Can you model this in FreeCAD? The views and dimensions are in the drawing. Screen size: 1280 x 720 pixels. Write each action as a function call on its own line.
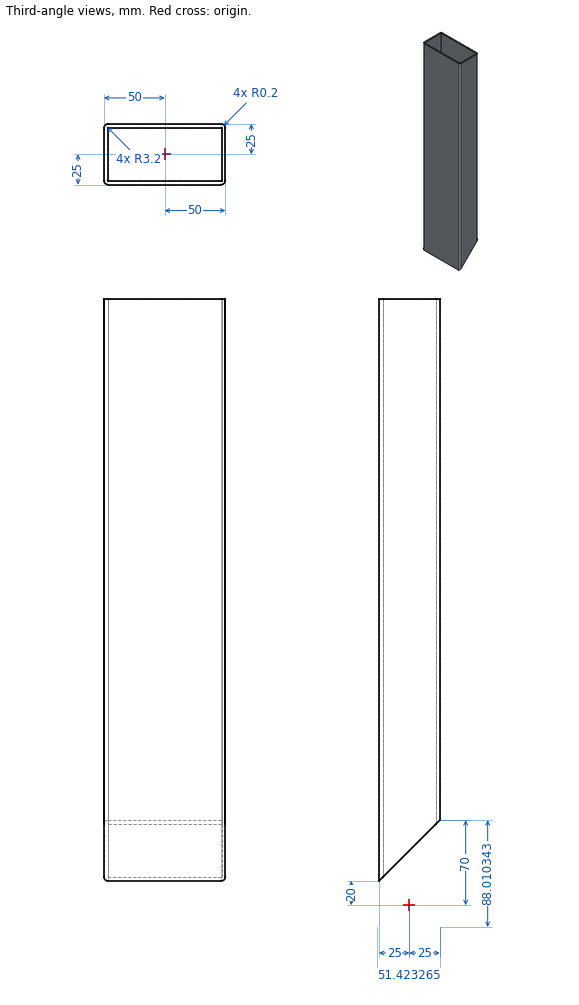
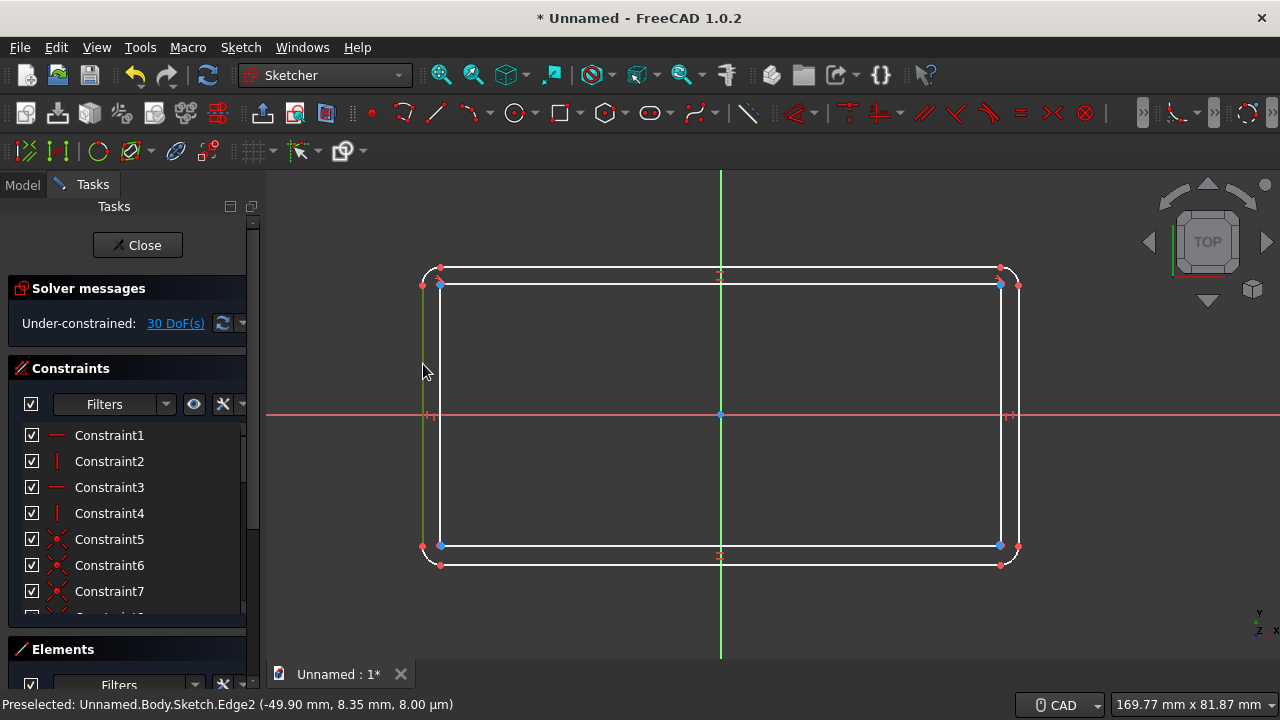
click(428, 272)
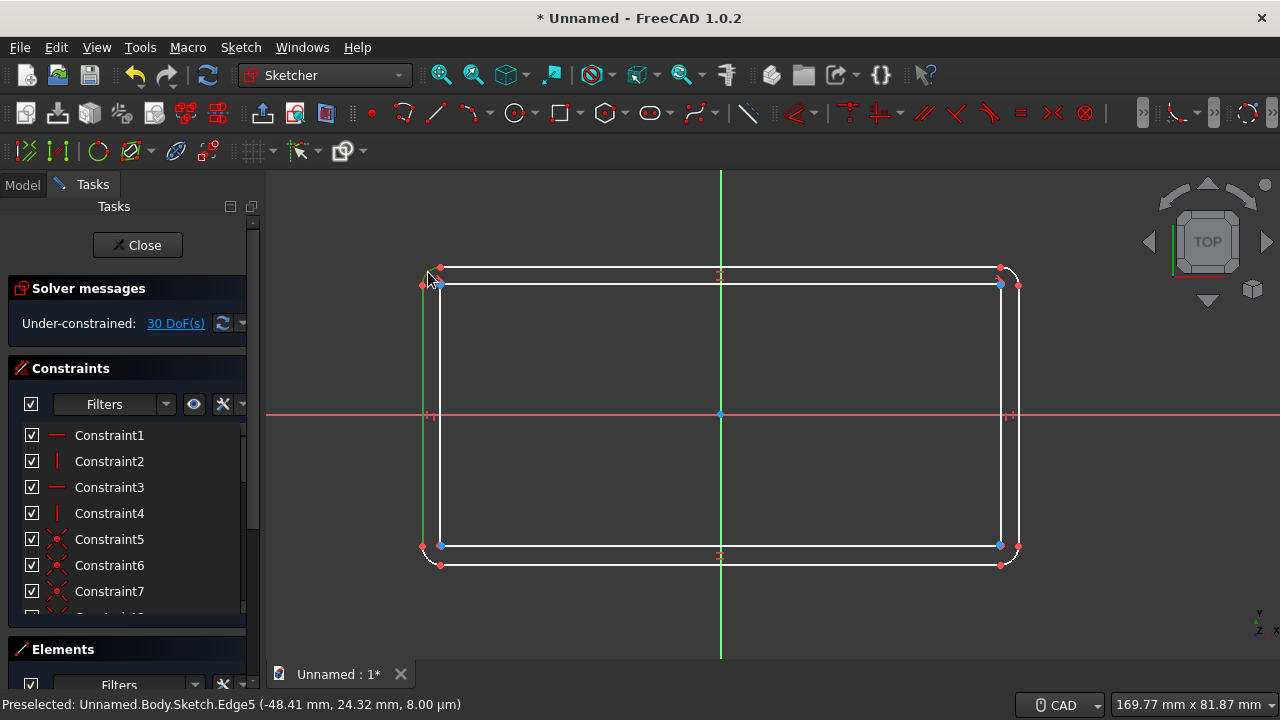
click(990, 114)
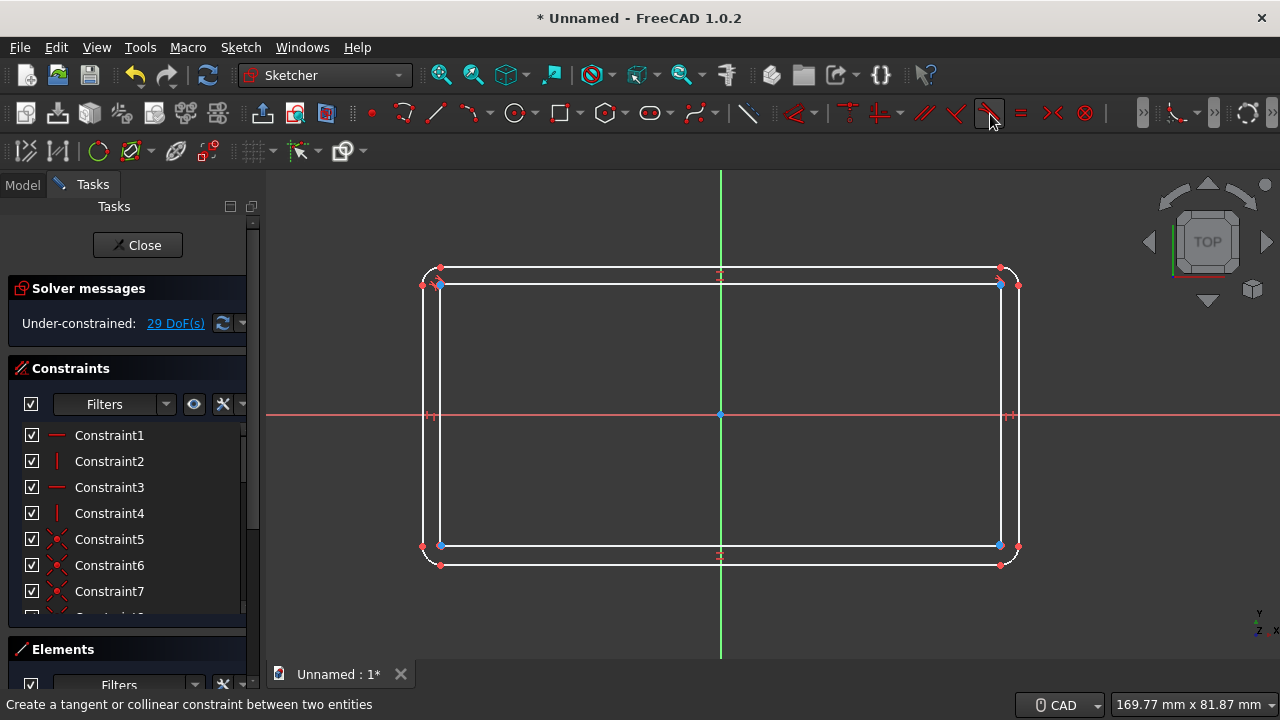
click(423, 364)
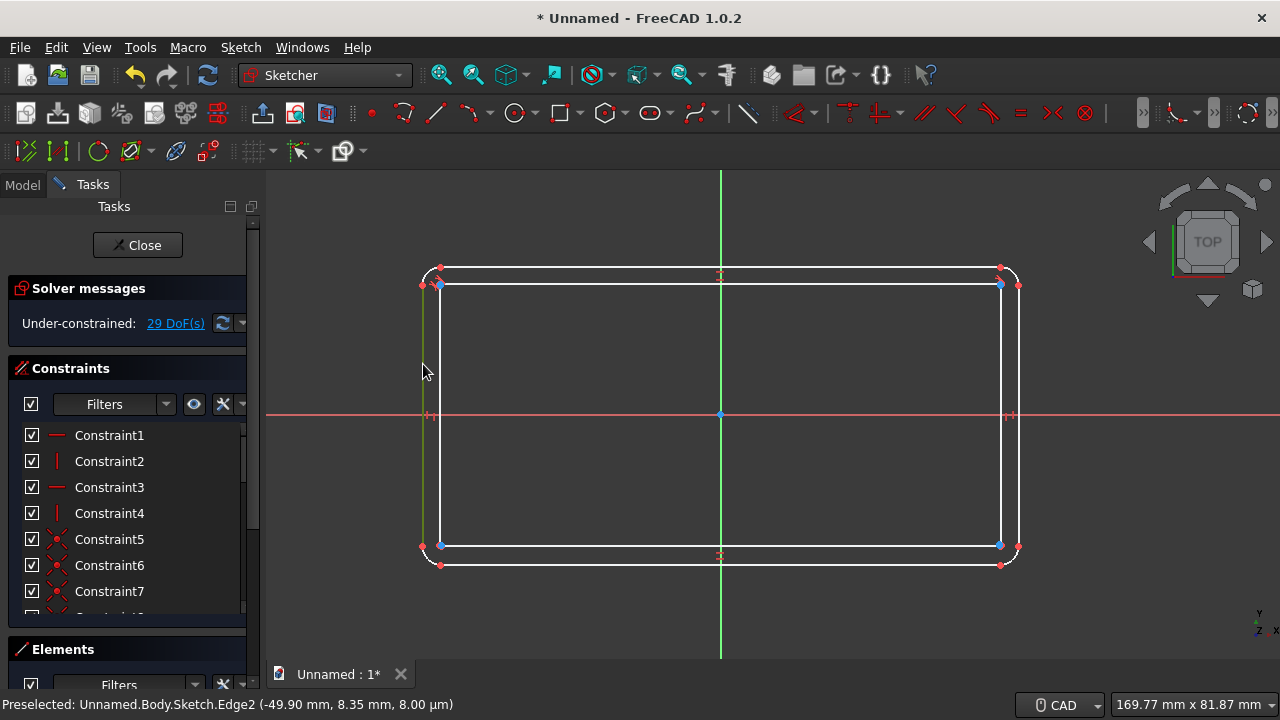
click(428, 559)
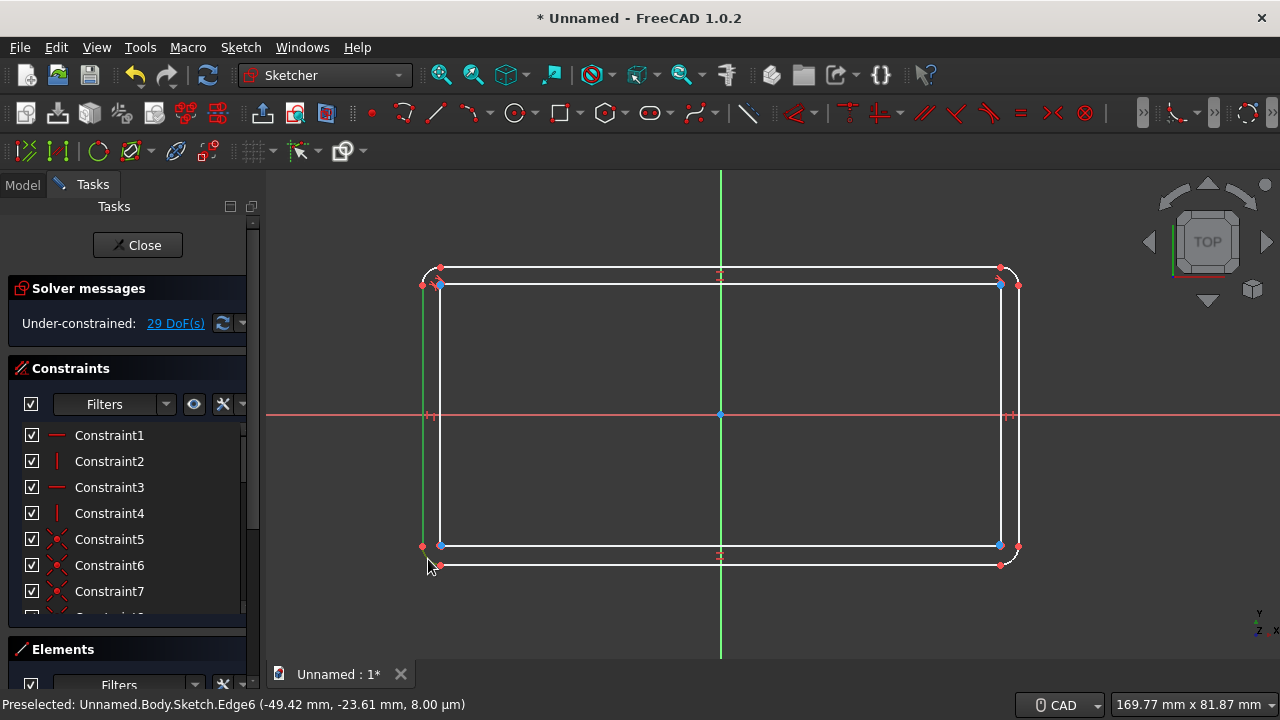
click(990, 114)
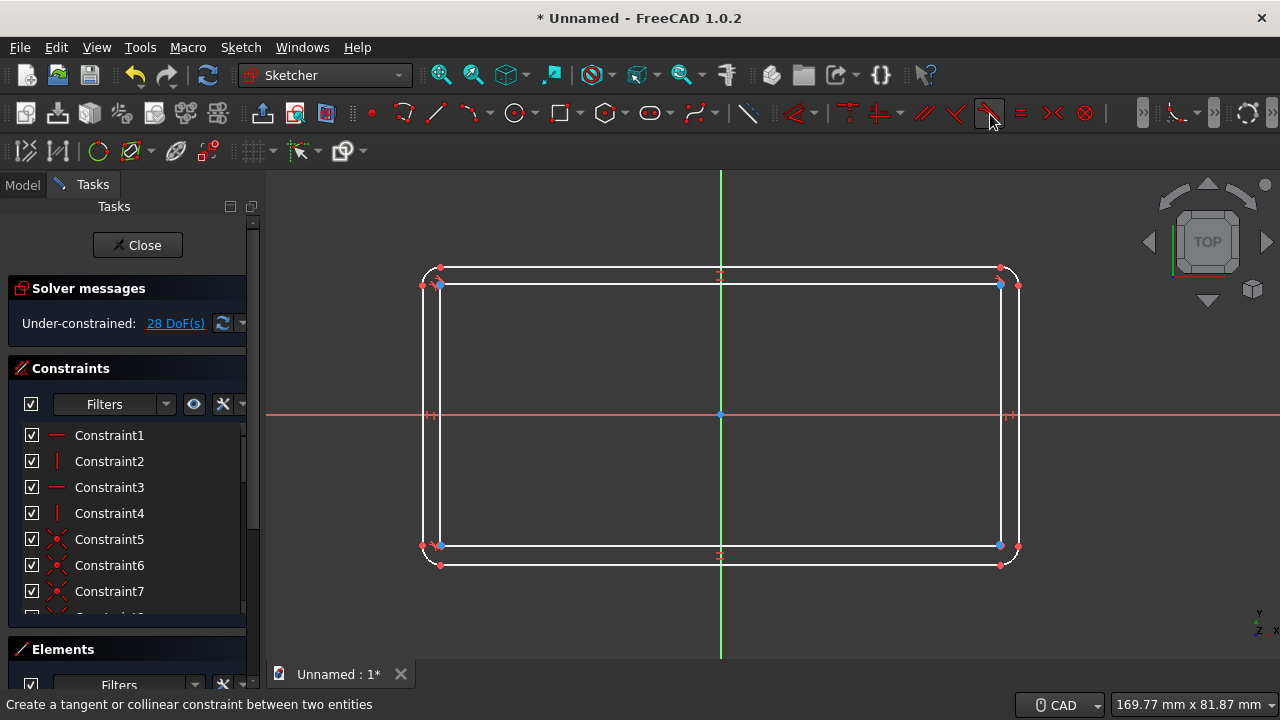
click(609, 565)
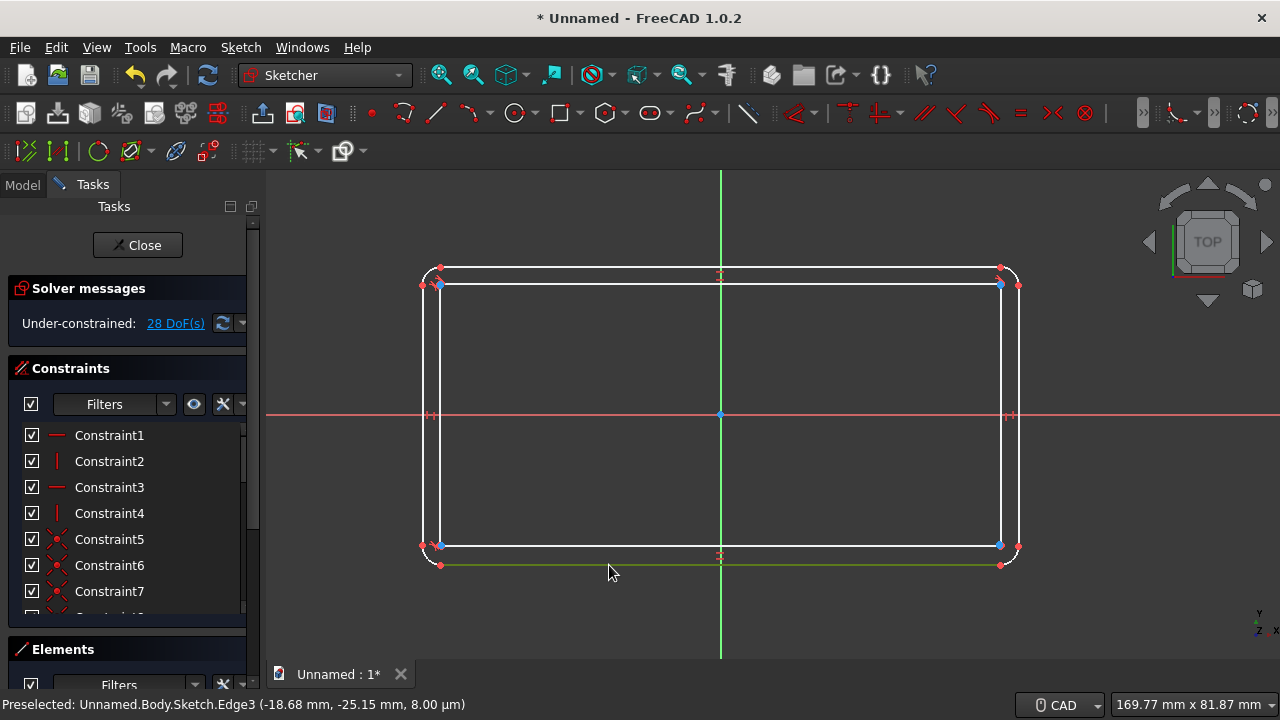
click(428, 559)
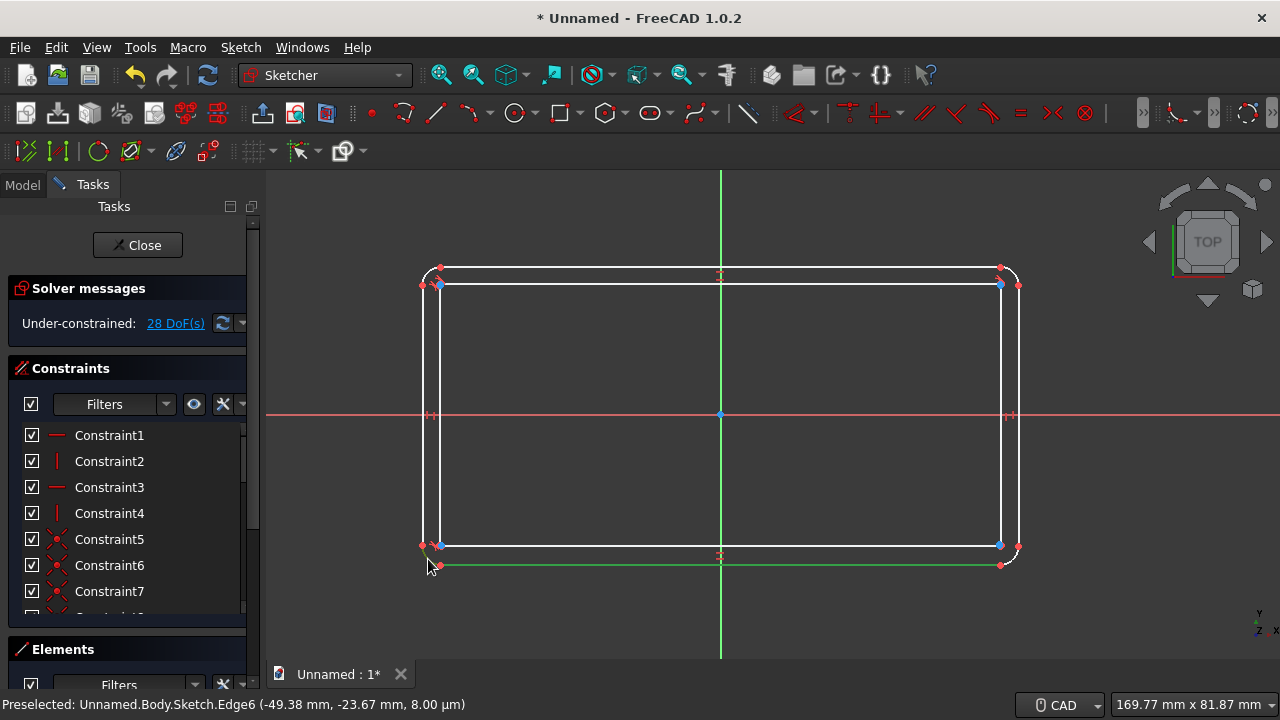
click(990, 114)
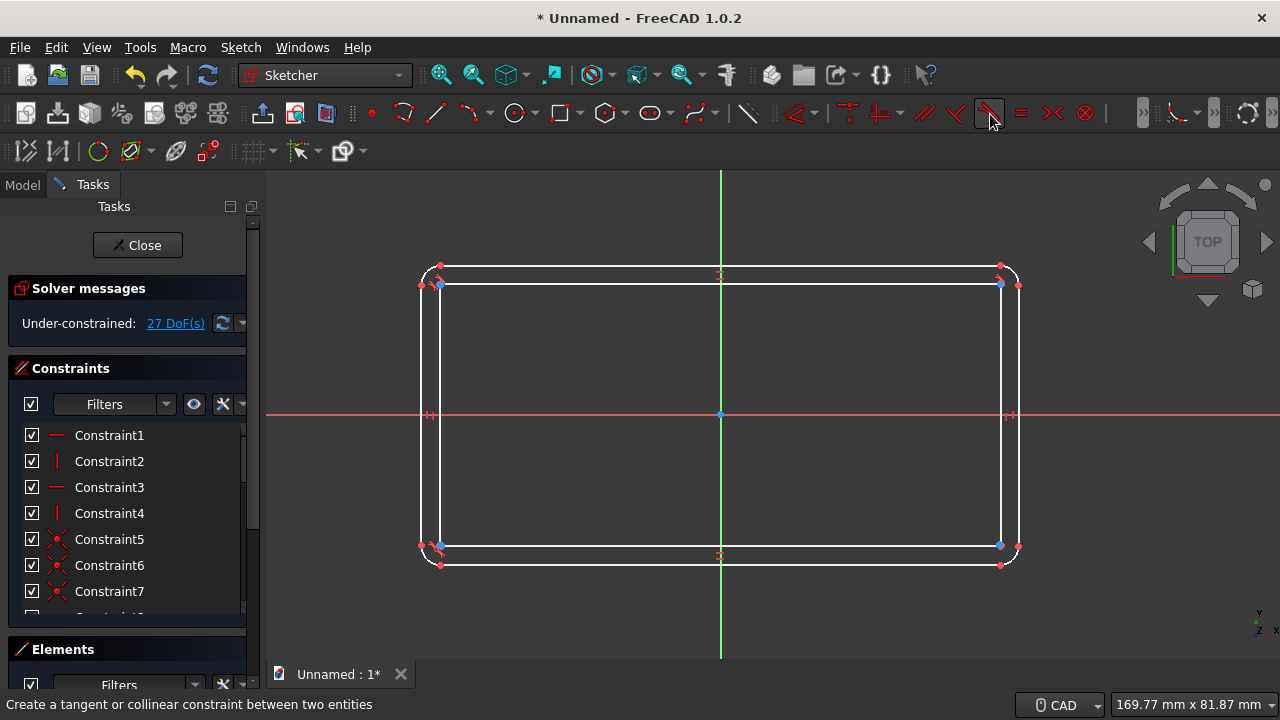
click(609, 565)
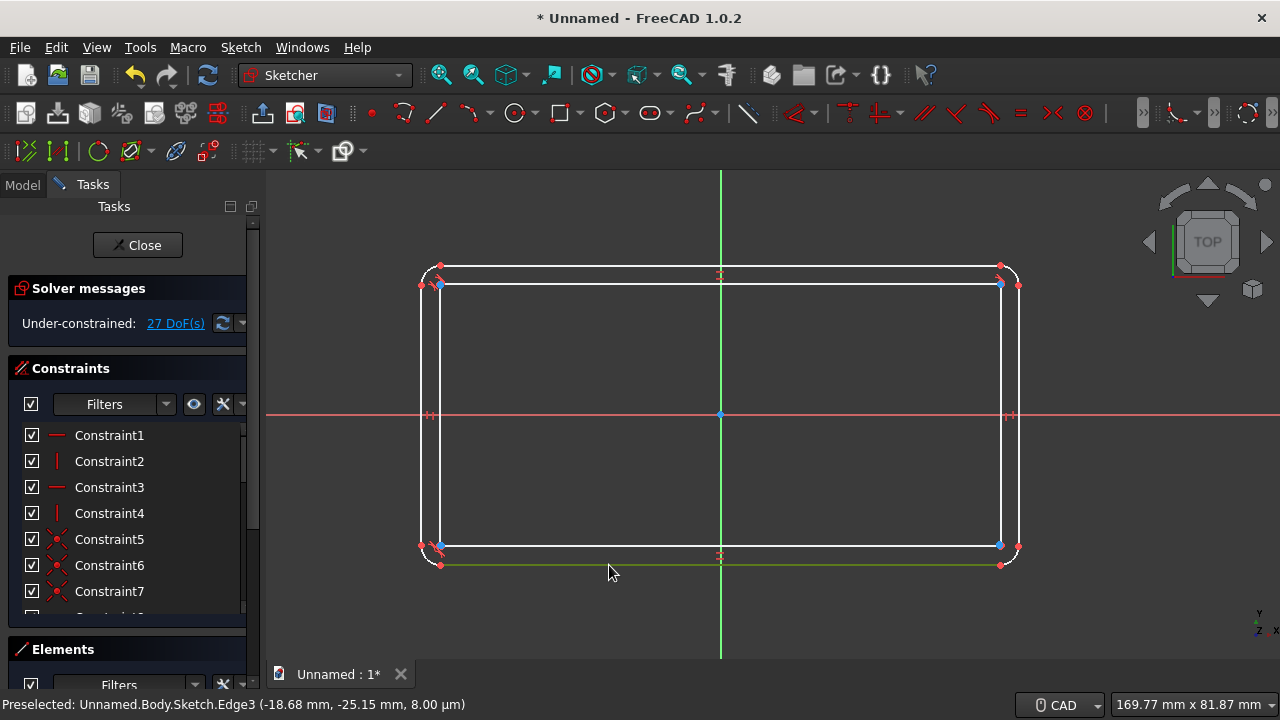
click(1013, 559)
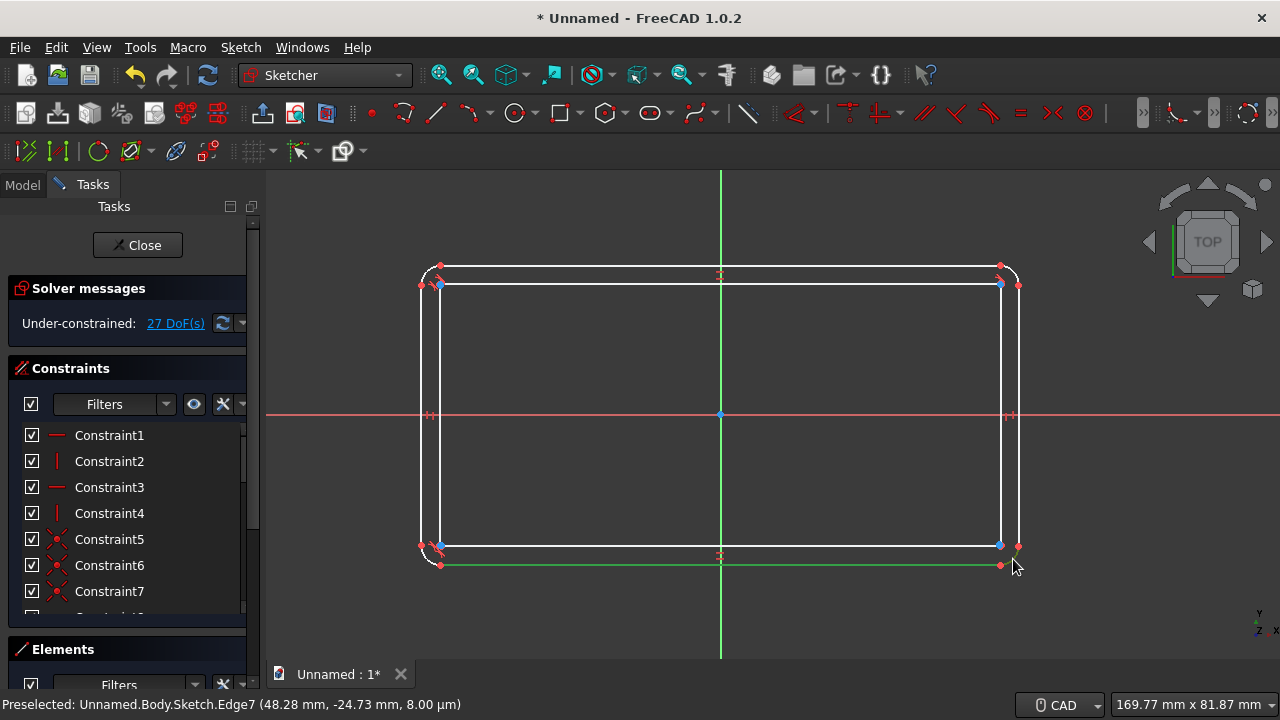
click(990, 114)